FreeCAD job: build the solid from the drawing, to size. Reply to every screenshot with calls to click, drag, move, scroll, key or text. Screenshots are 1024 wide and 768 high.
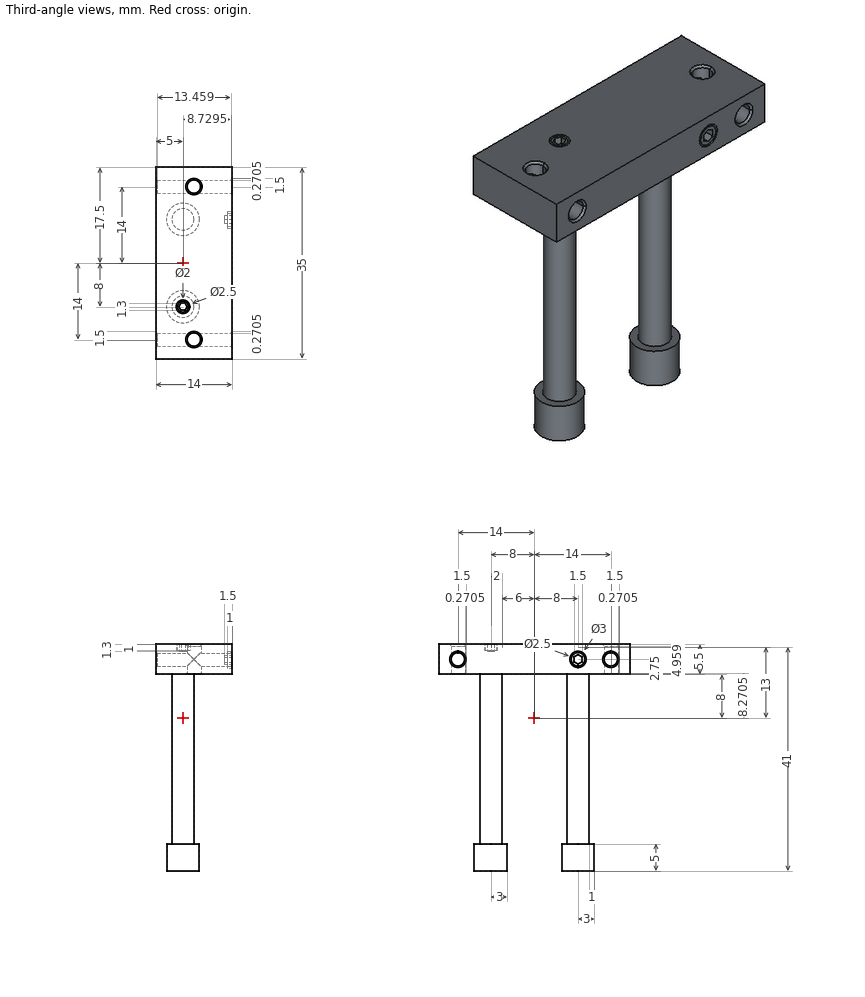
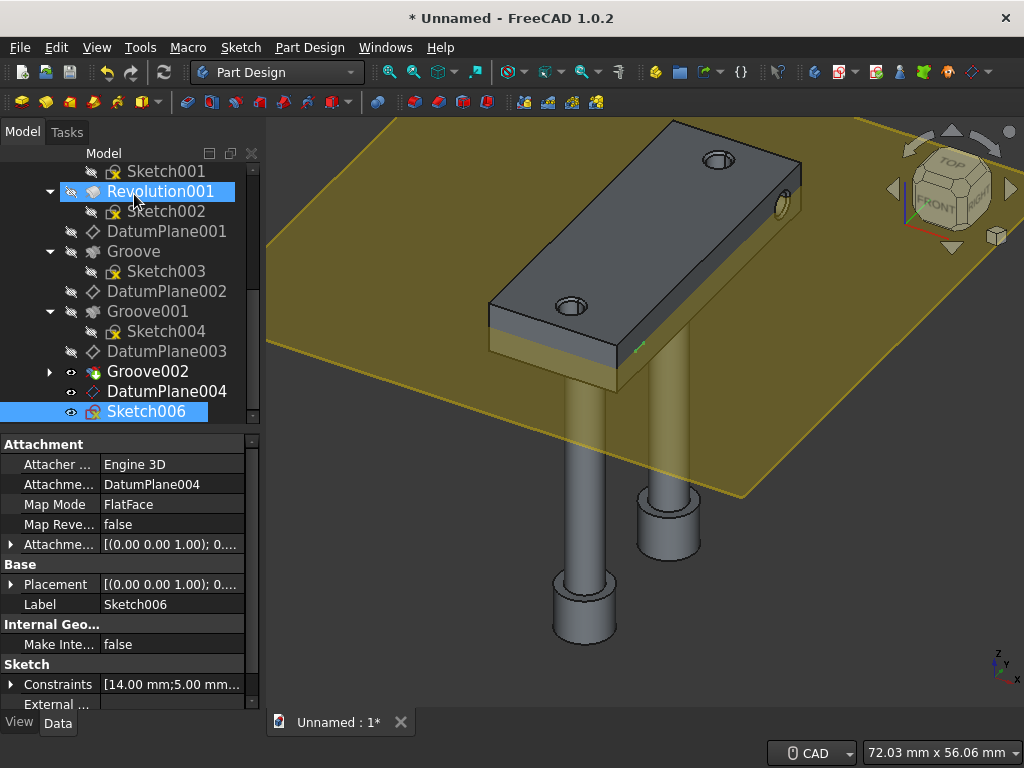
click(236, 102)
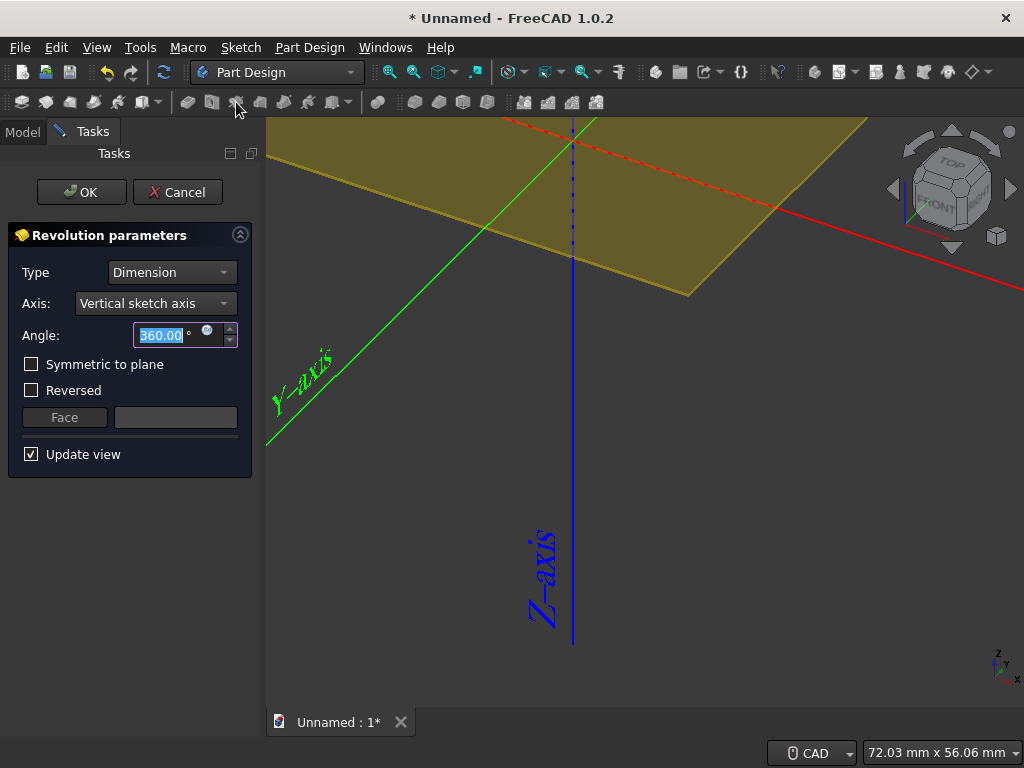
click(156, 304)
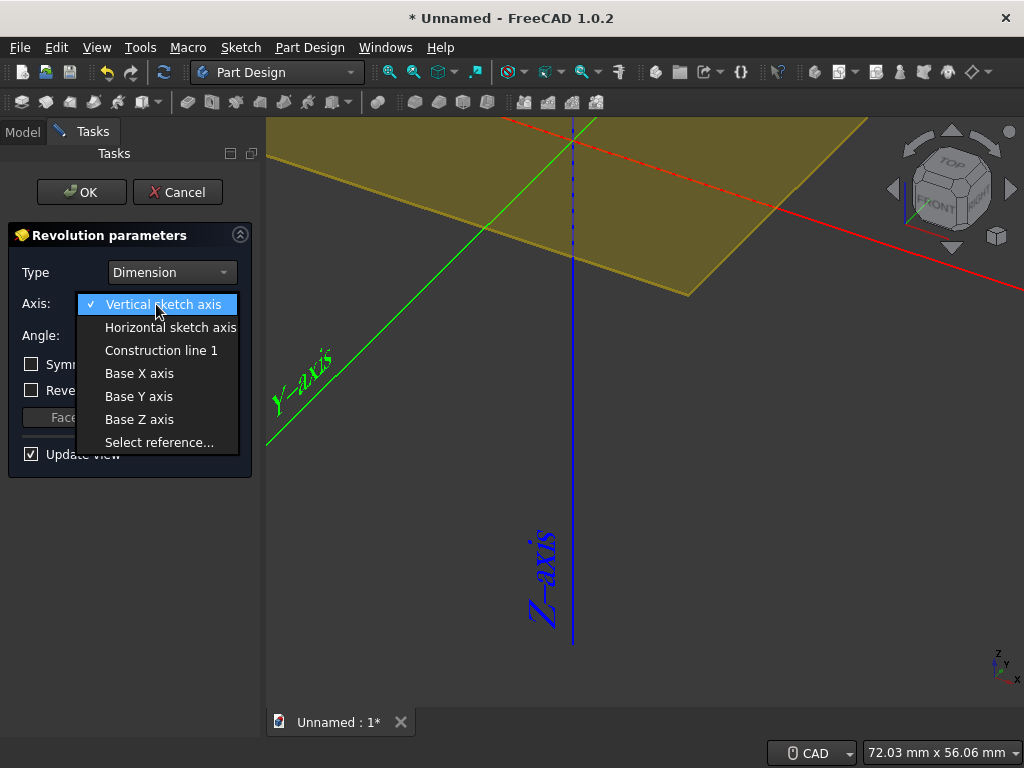
click(156, 350)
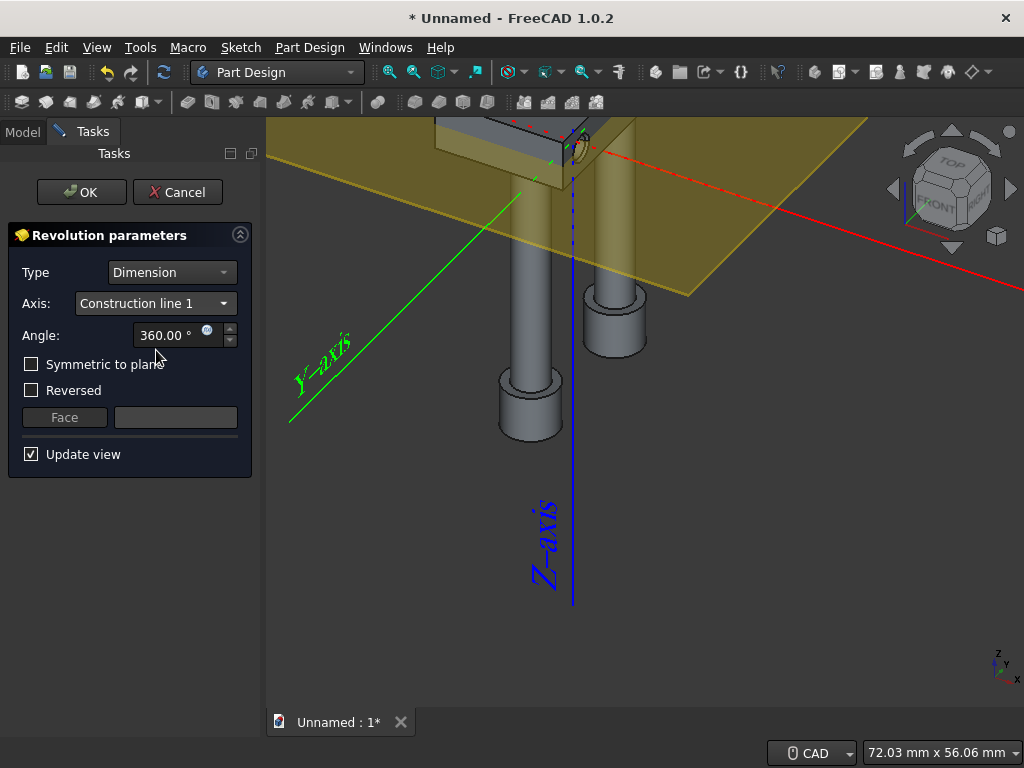
click(82, 192)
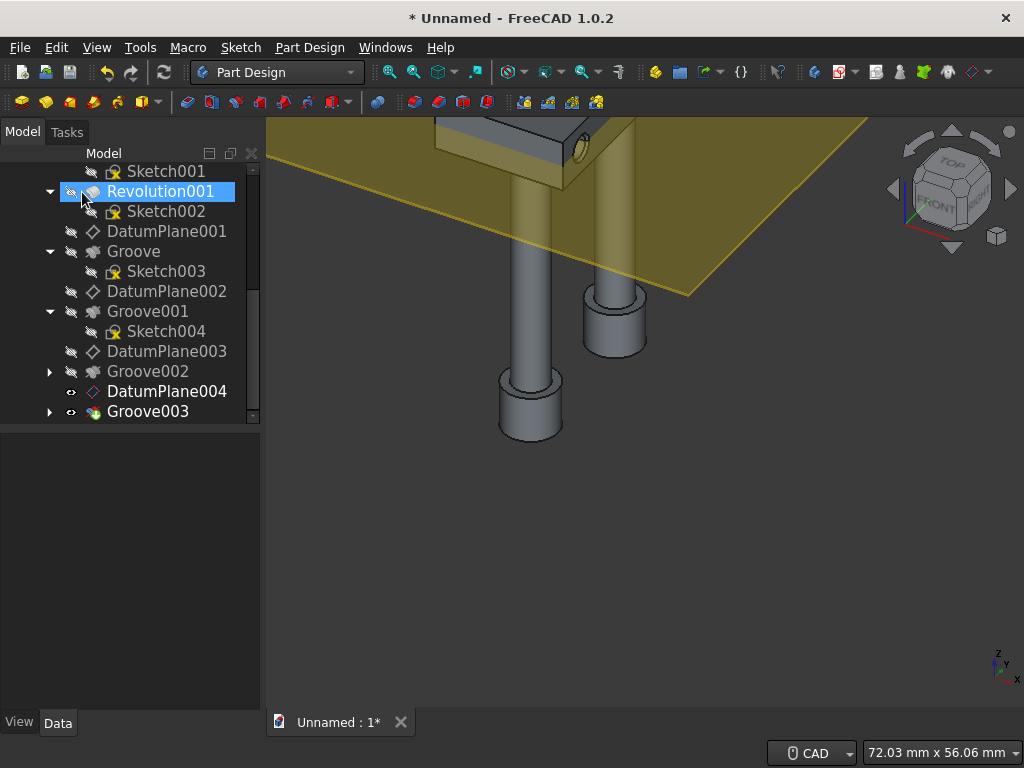
click(116, 392)
key(space)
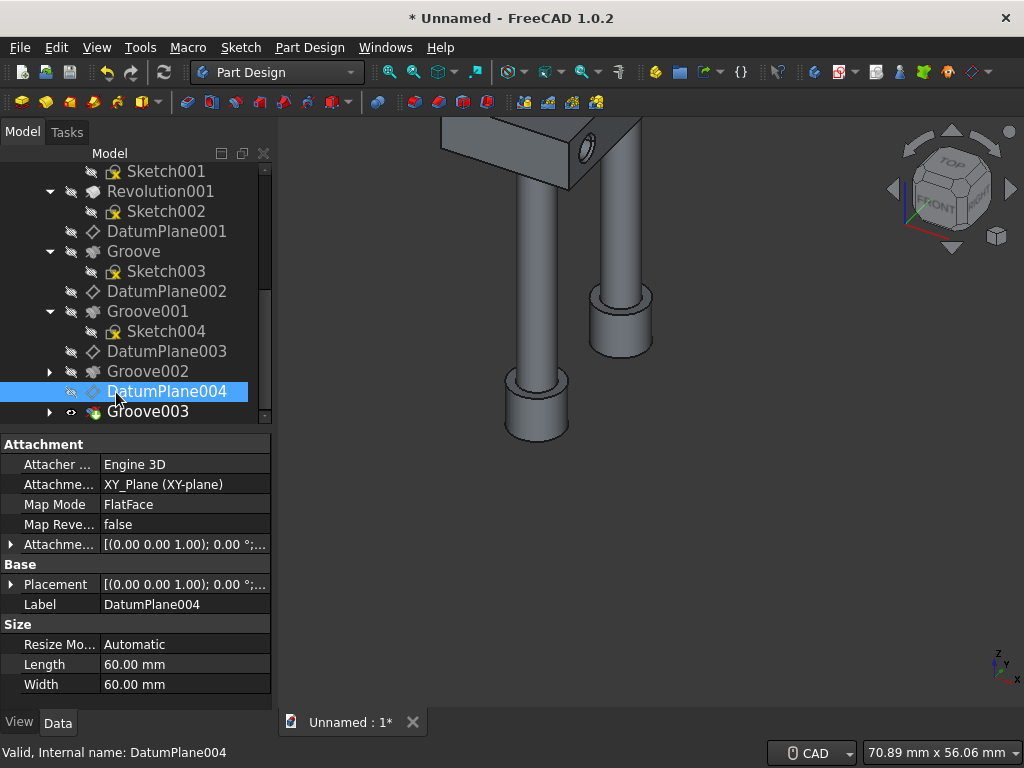
click(390, 72)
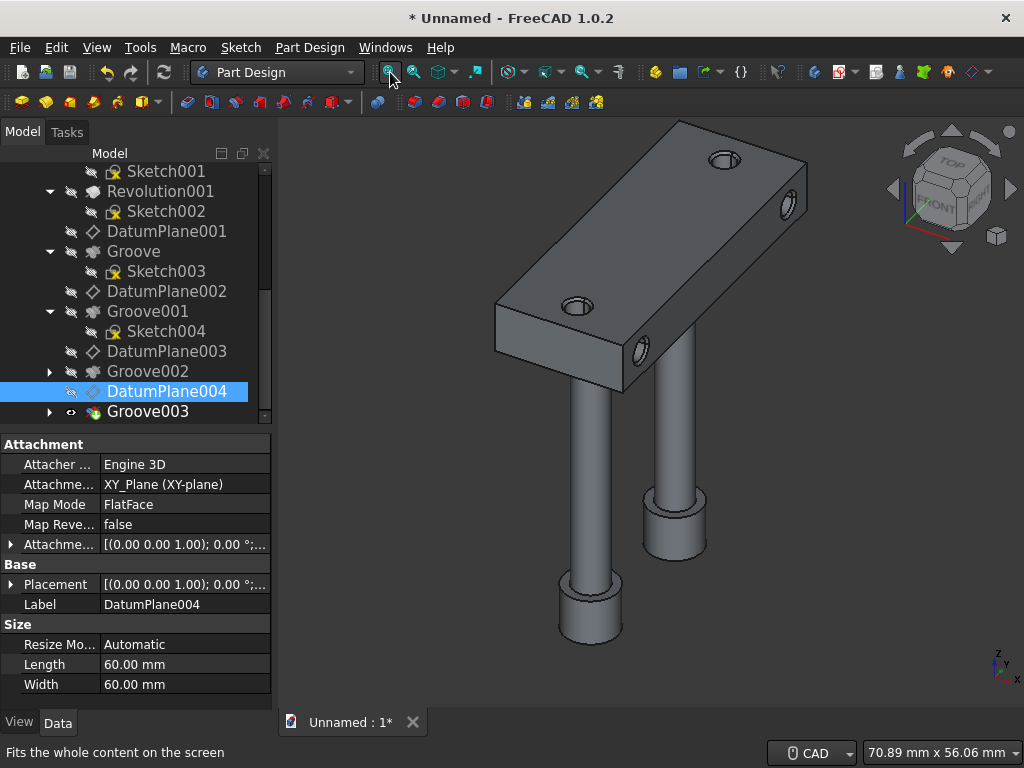
click(677, 206)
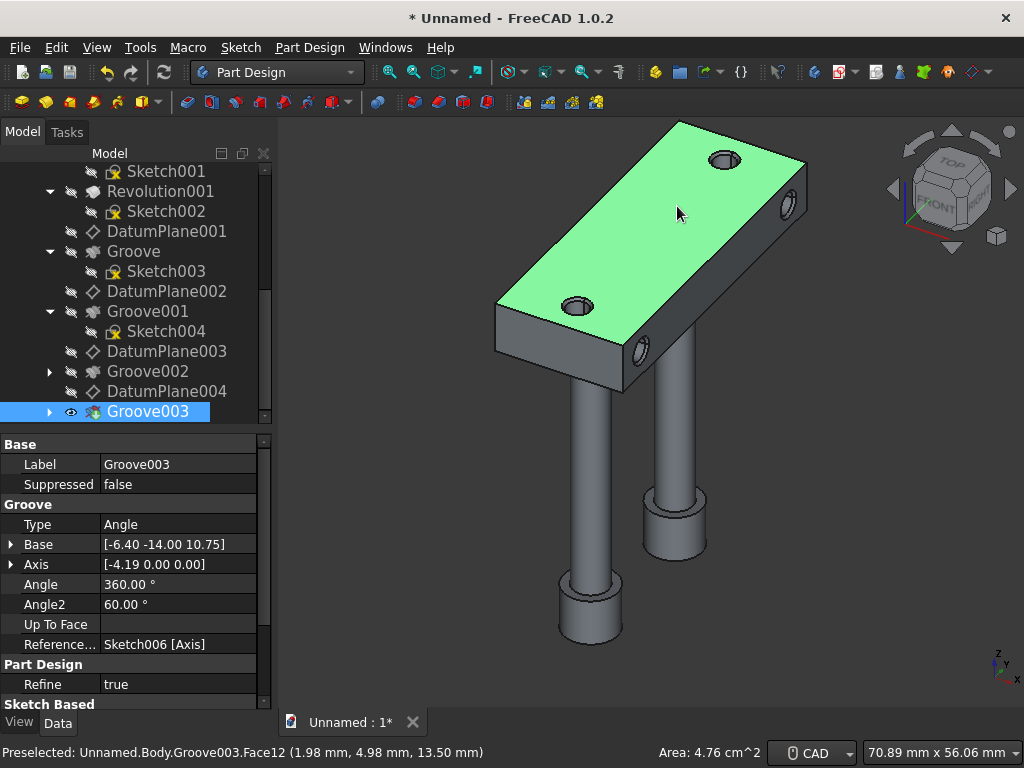
click(840, 72)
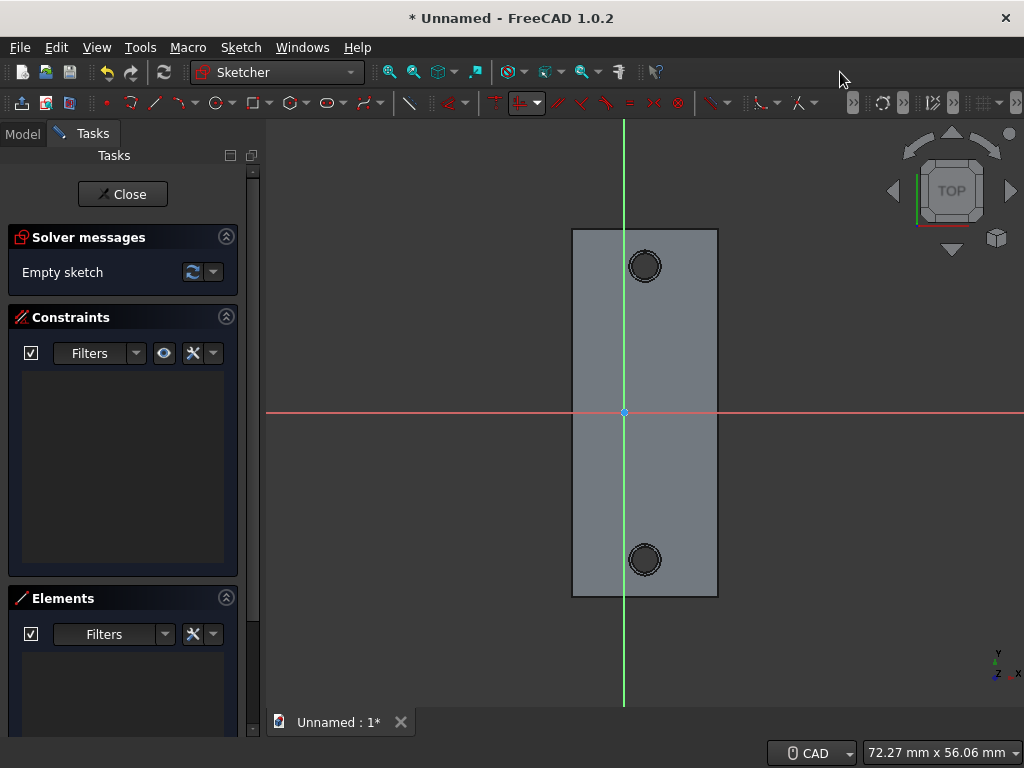
scroll(628, 504, up, 13)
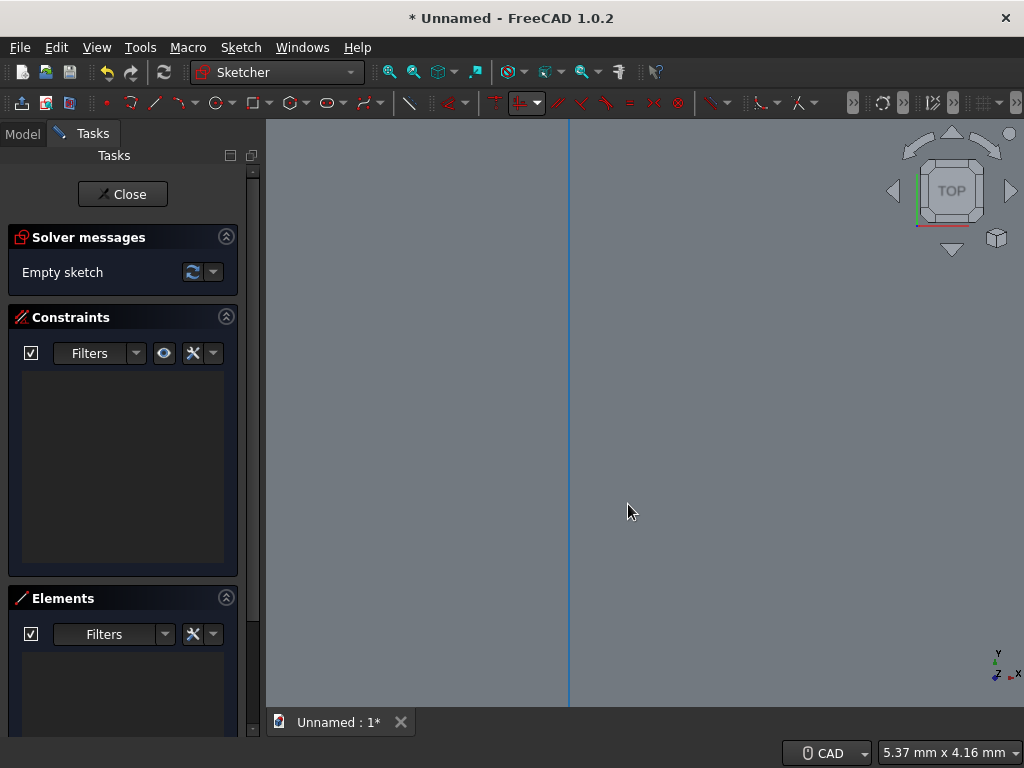
click(216, 104)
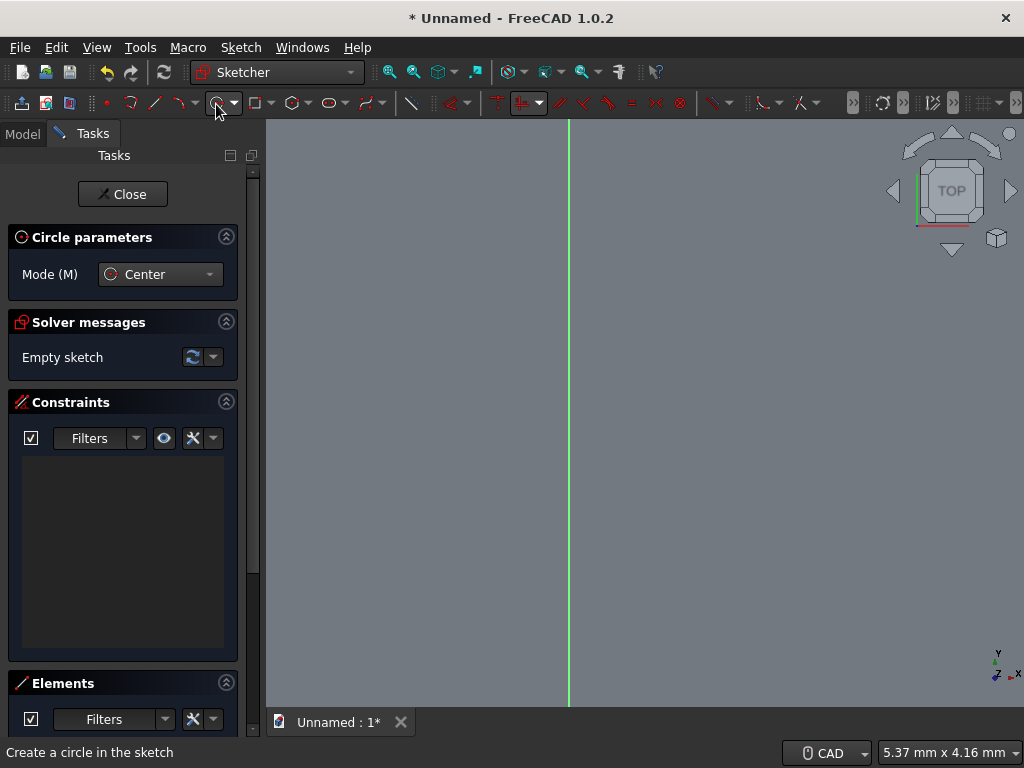
click(569, 400)
move(693, 275)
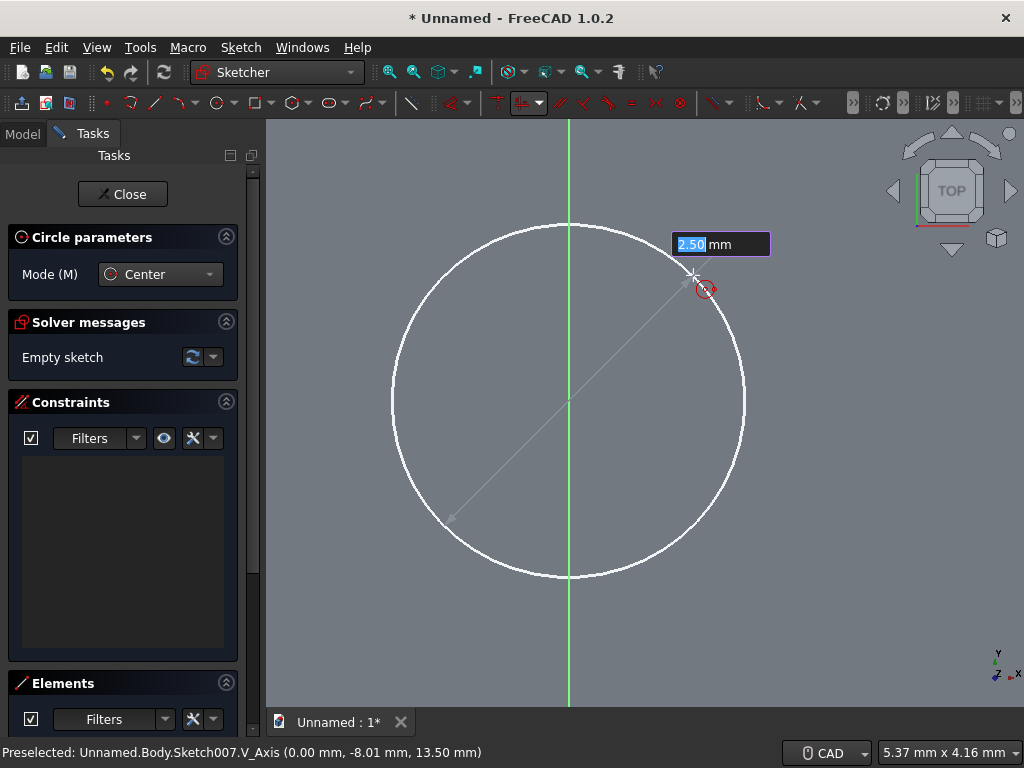
text(2.5)
key(Return)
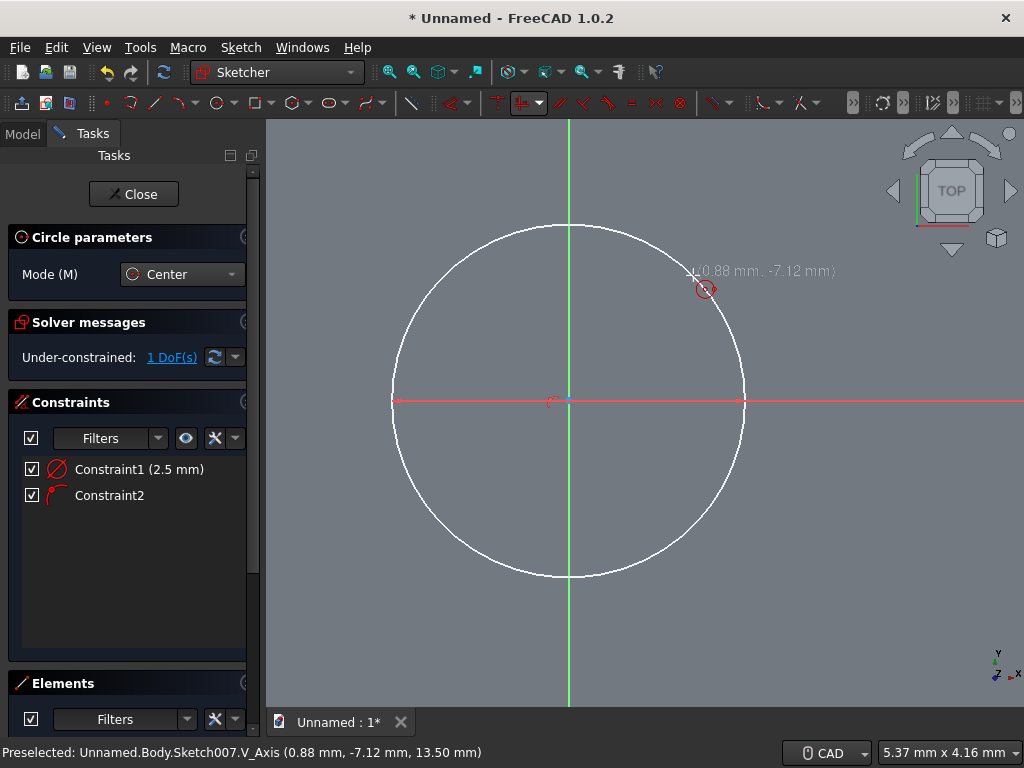
click(569, 401)
move(668, 300)